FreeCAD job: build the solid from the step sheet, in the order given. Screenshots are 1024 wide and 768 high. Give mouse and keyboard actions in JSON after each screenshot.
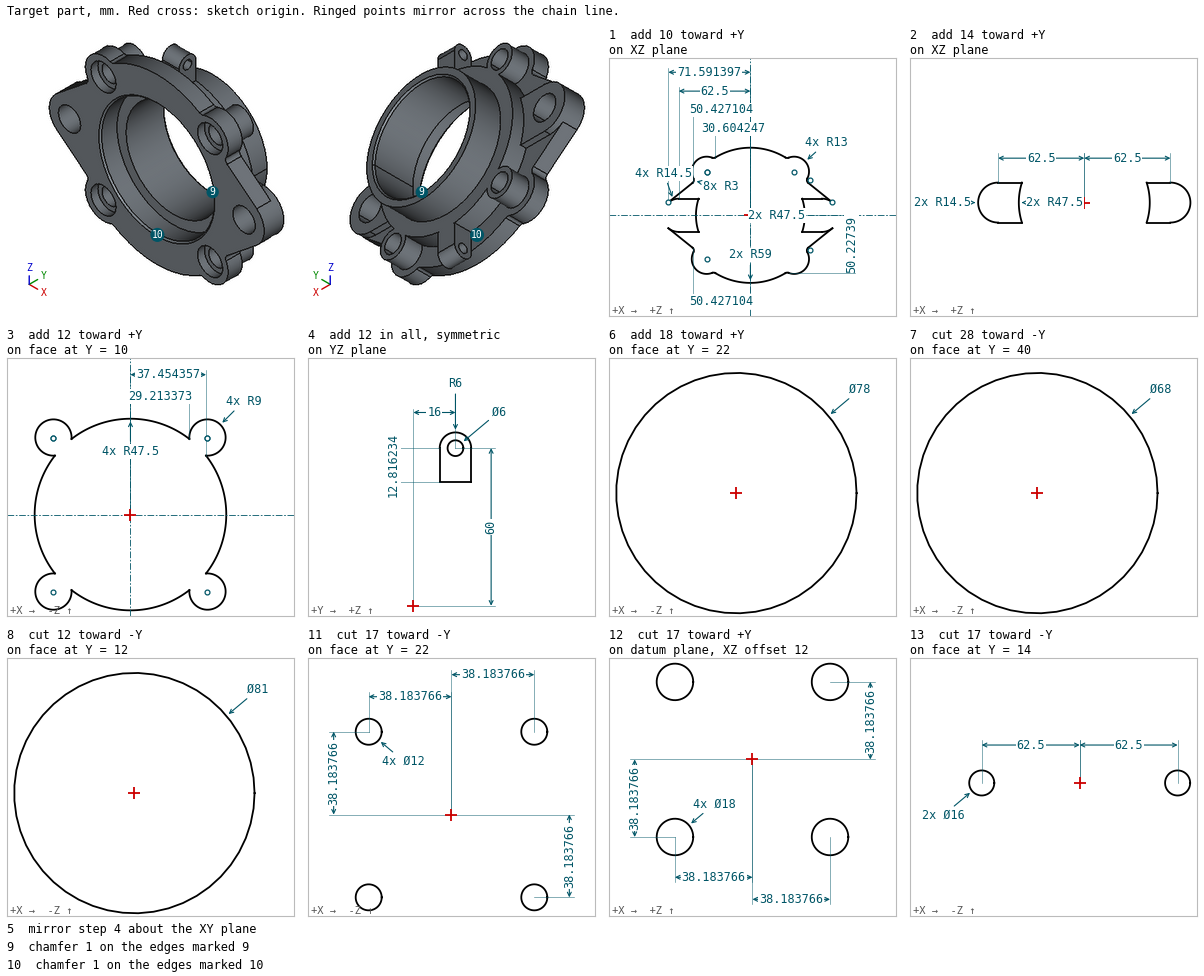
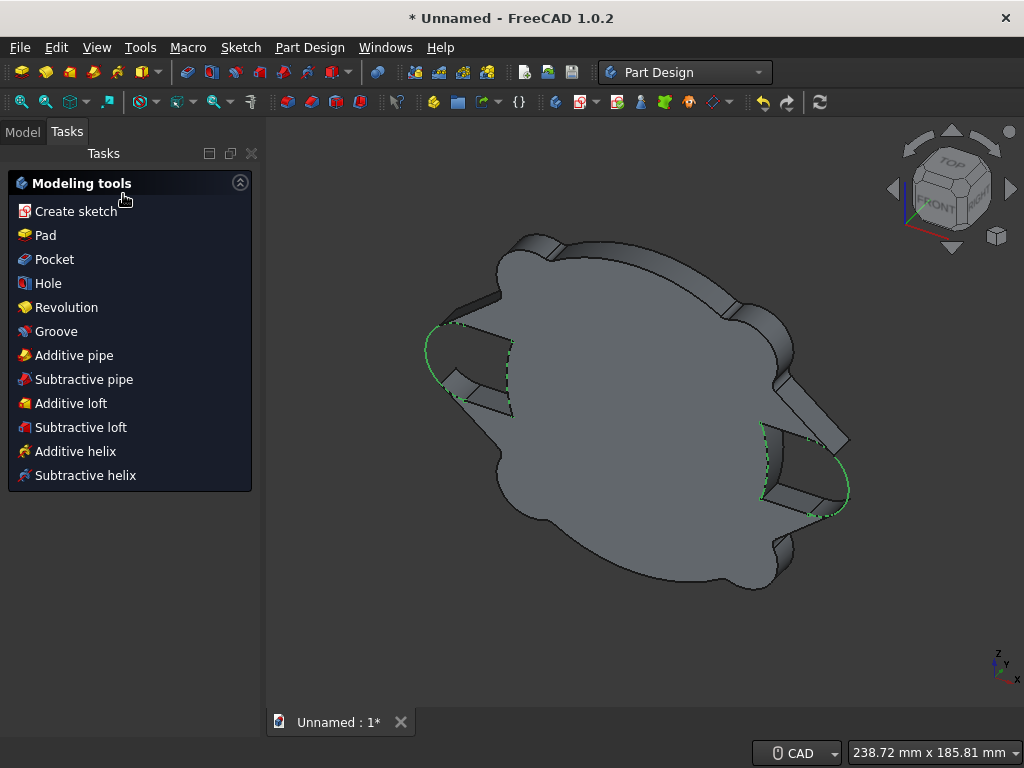
{"action": "left_click", "coordinate": [22, 72]}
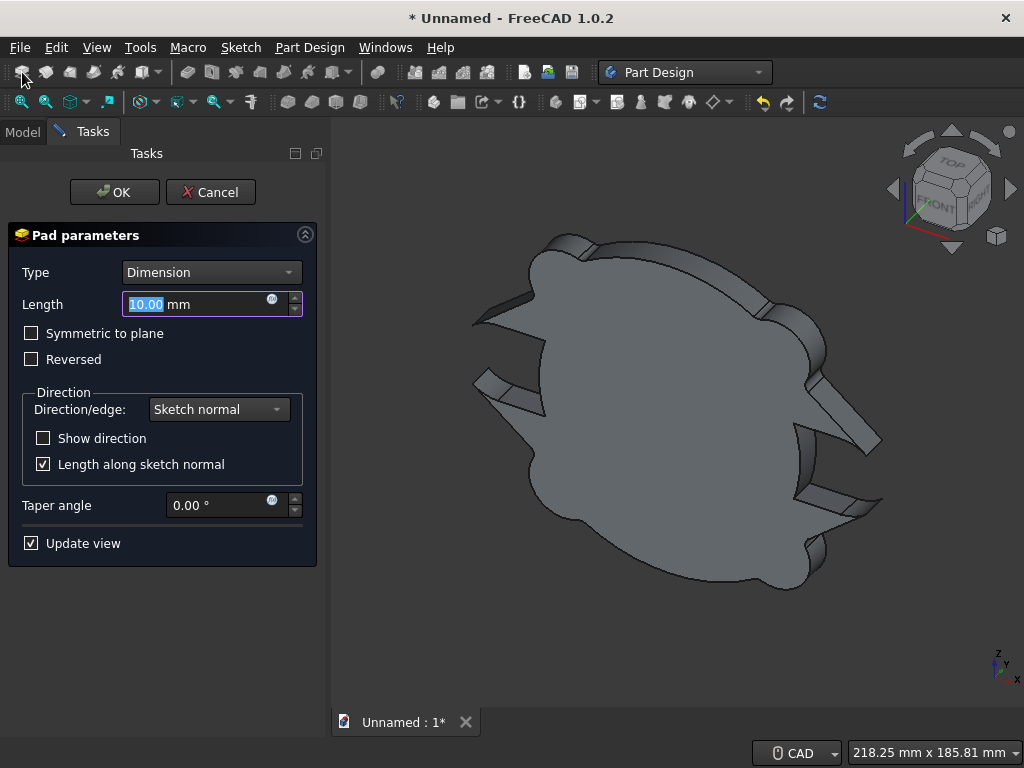
{"action": "type", "text": "14"}
{"action": "key", "text": "Tab"}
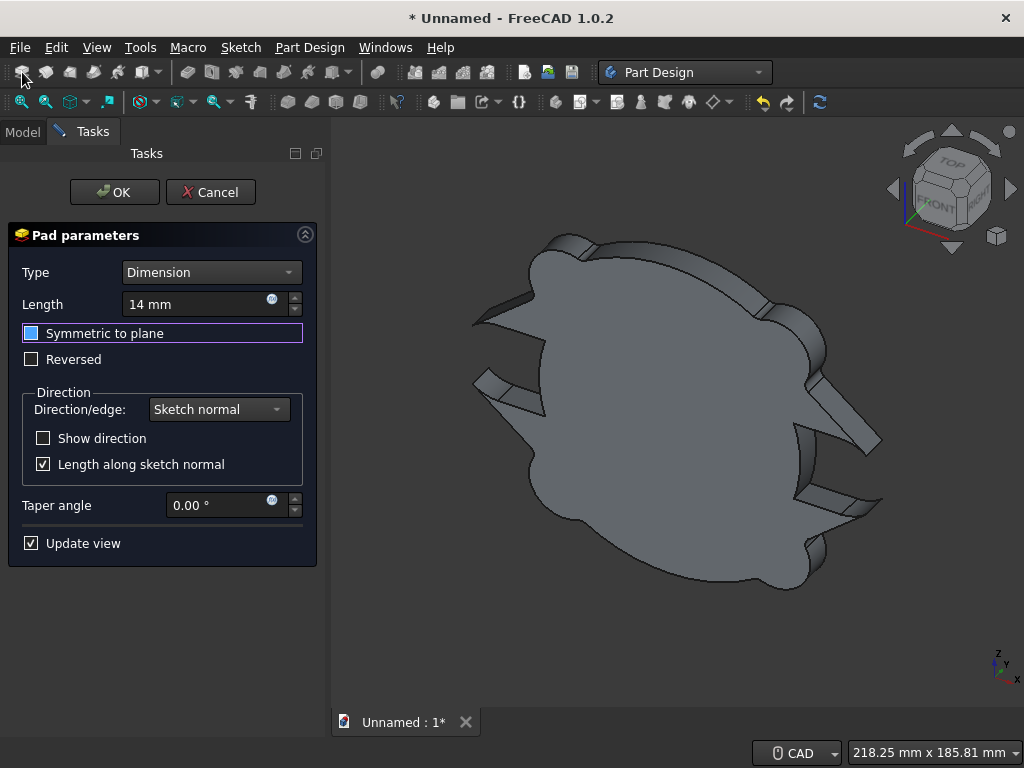
{"action": "left_click", "coordinate": [30, 359]}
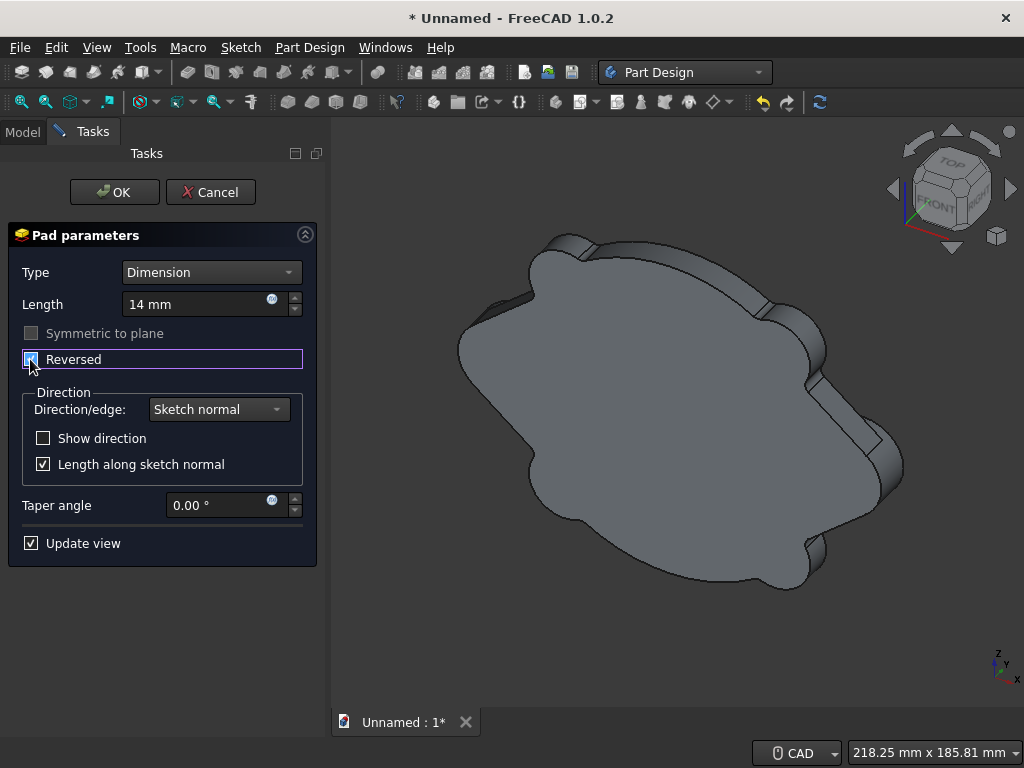
{"action": "left_click", "coordinate": [115, 192]}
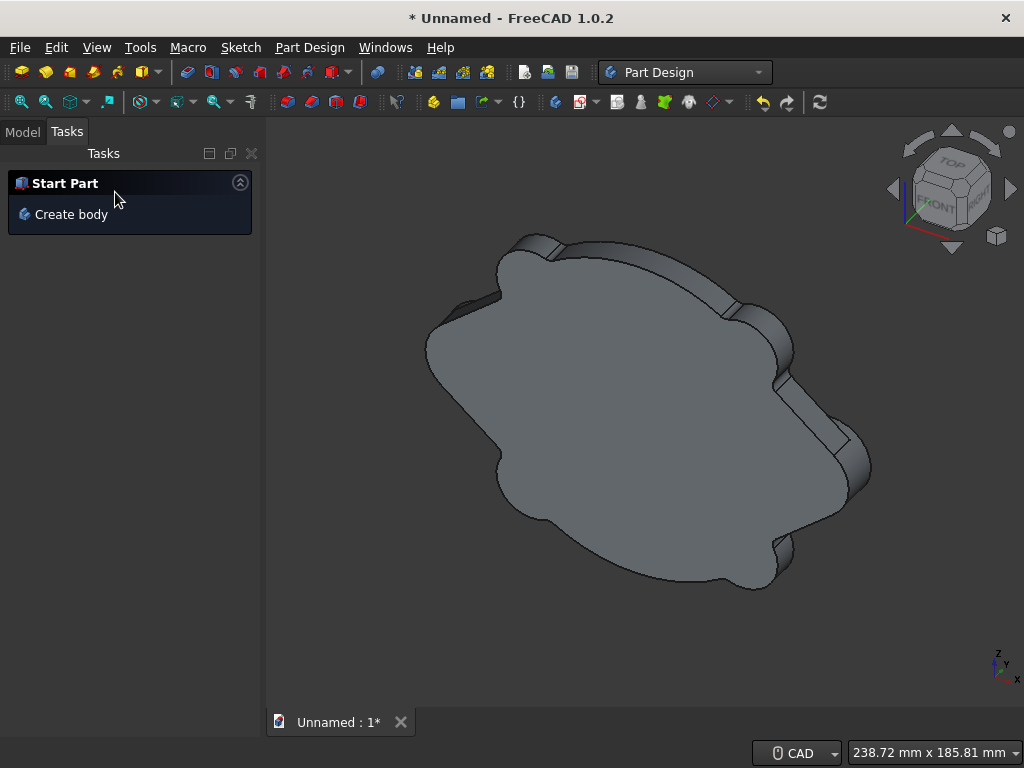
{"action": "key", "text": "4"}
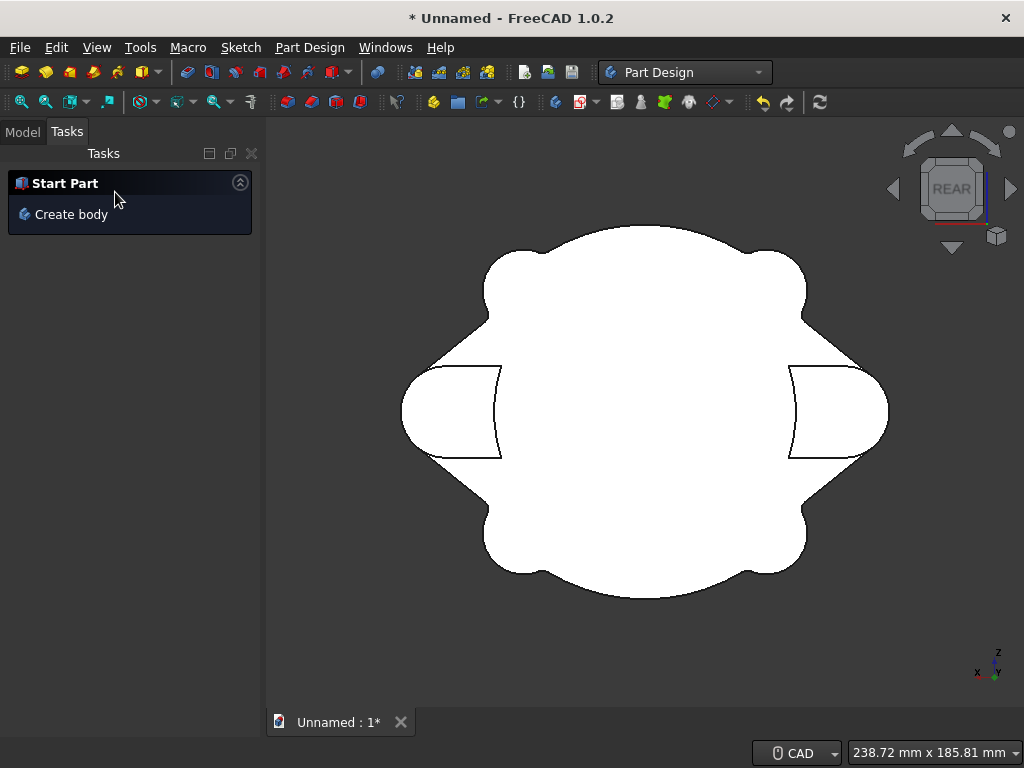
{"action": "left_click", "coordinate": [645, 411]}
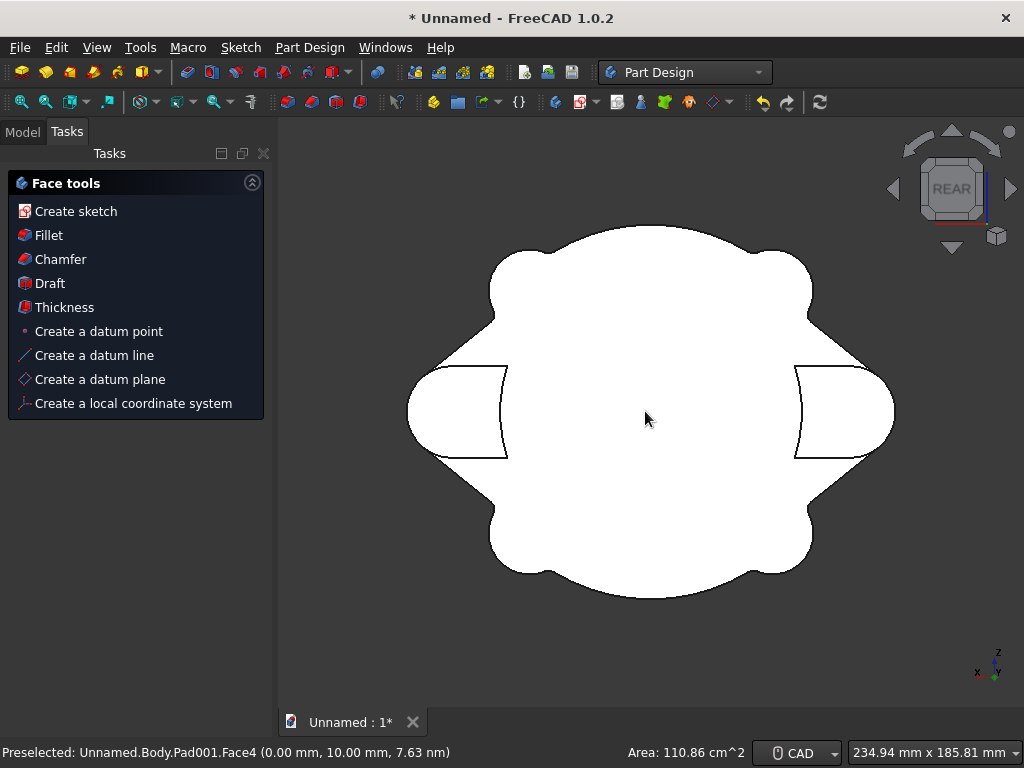
{"action": "left_click", "coordinate": [580, 102]}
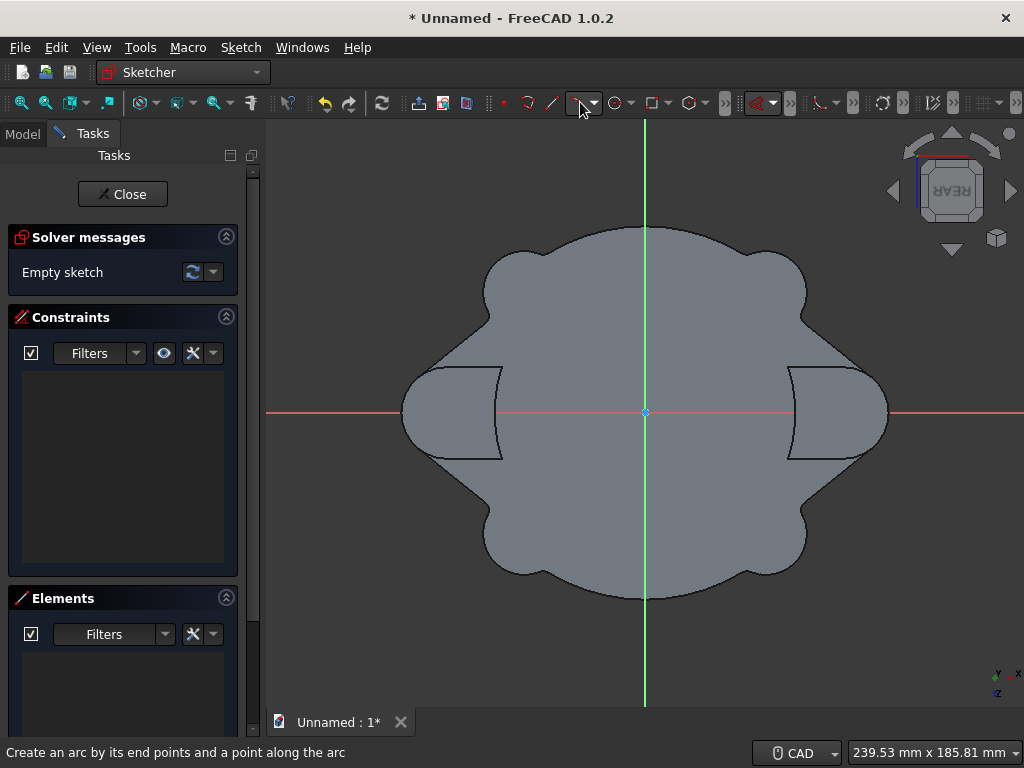
{"action": "left_click", "coordinate": [468, 104]}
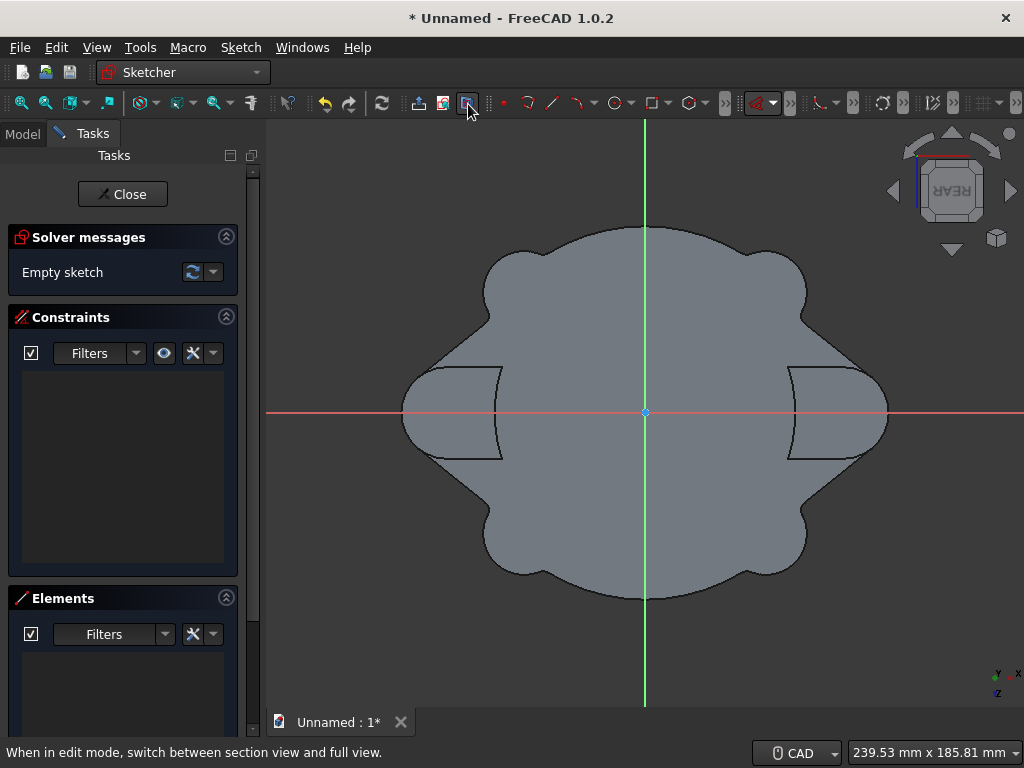
{"action": "left_click", "coordinate": [578, 104]}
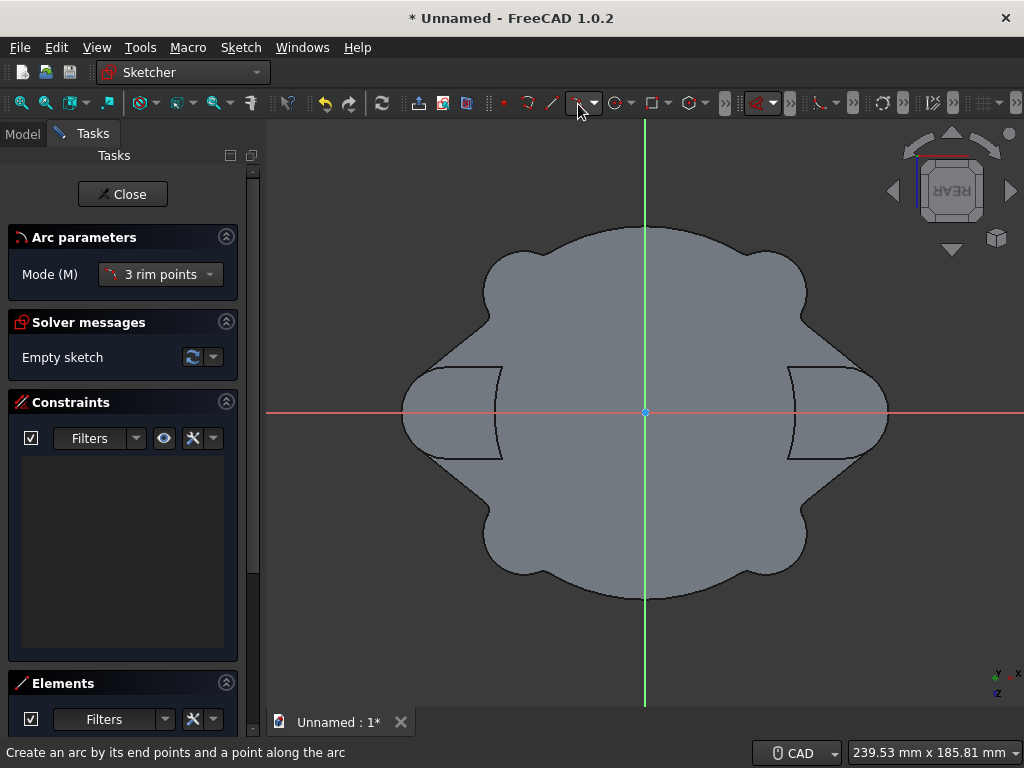
{"action": "left_click", "coordinate": [764, 321]}
{"action": "left_click", "coordinate": [737, 294]}
{"action": "left_click", "coordinate": [786, 272]}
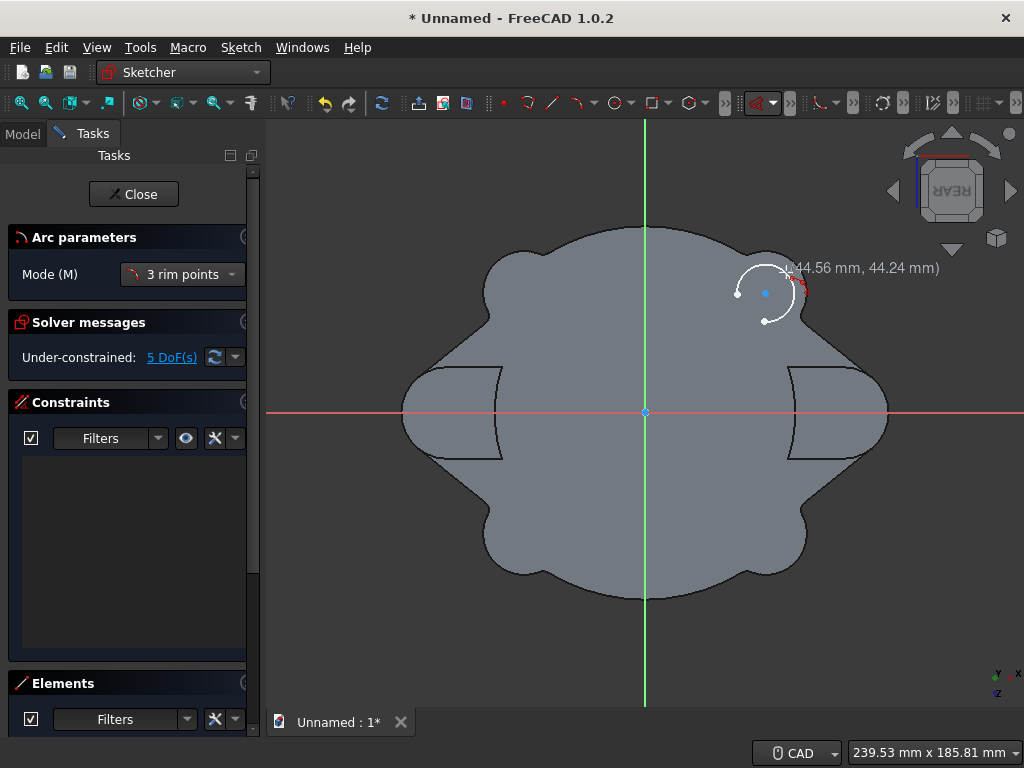
{"action": "left_click", "coordinate": [737, 295]}
{"action": "left_click", "coordinate": [553, 294]}
{"action": "left_click", "coordinate": [665, 264]}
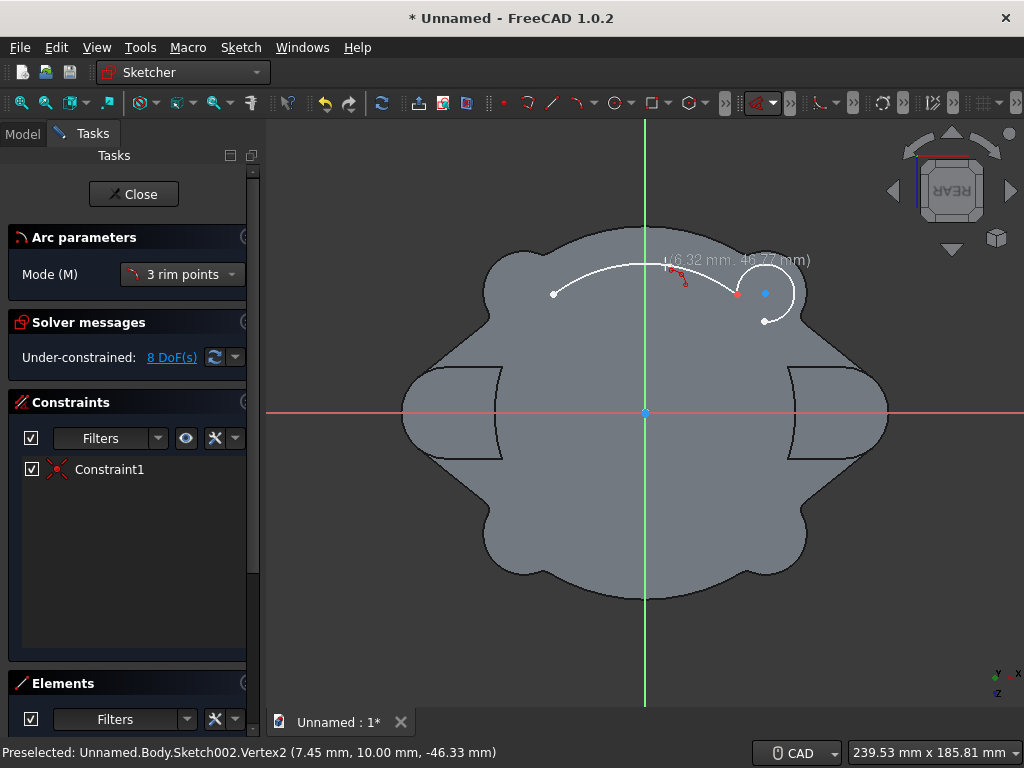
{"action": "left_click", "coordinate": [553, 295]}
{"action": "left_click", "coordinate": [526, 321]}
{"action": "left_click", "coordinate": [504, 272]}